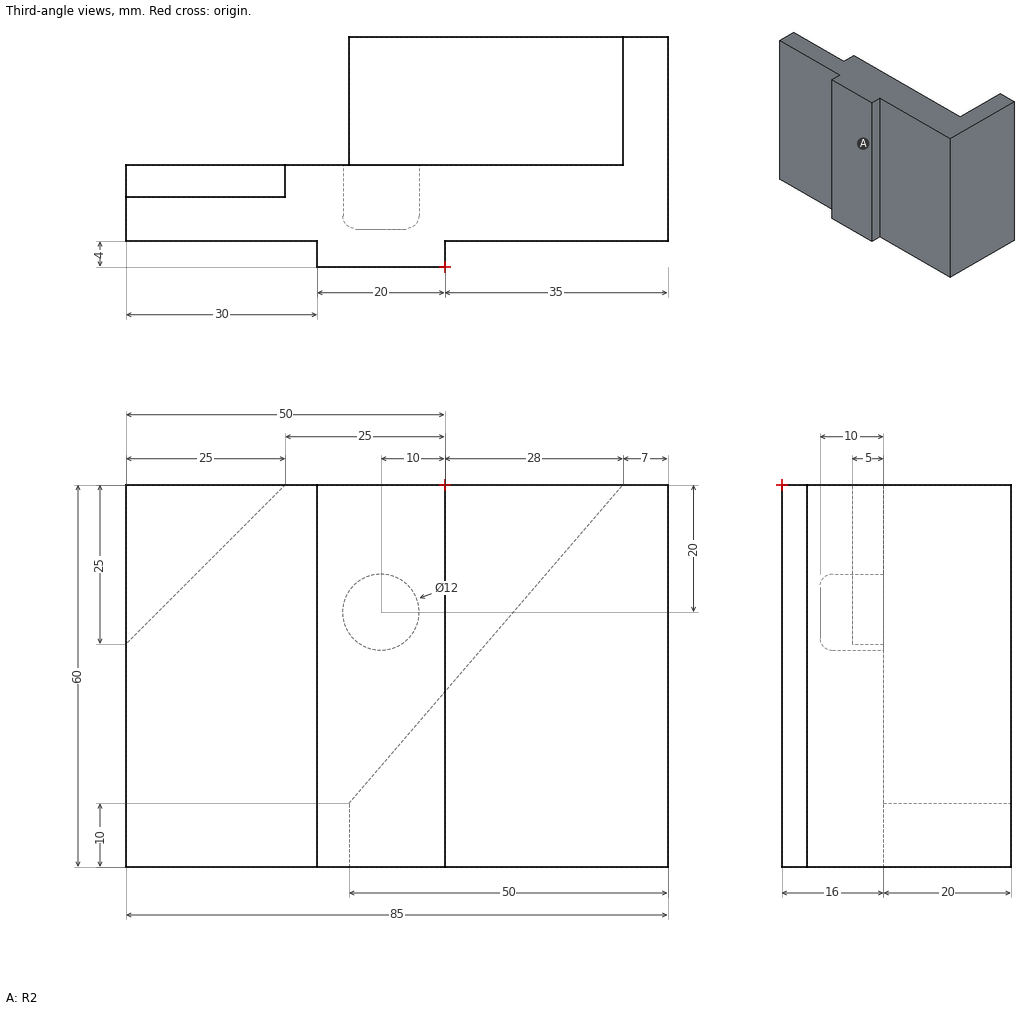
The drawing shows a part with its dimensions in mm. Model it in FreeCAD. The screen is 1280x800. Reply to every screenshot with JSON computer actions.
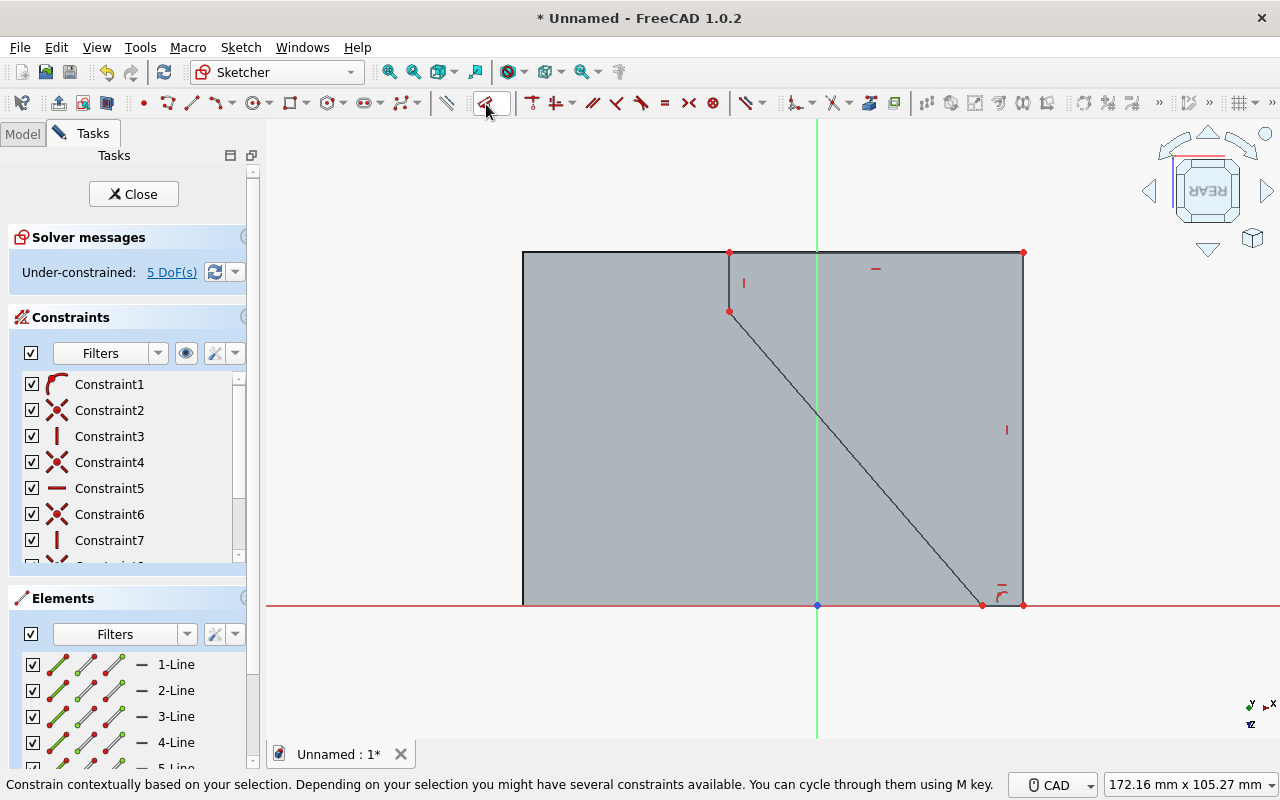
{"action": "left_click", "coordinate": [994, 606]}
{"action": "left_click", "coordinate": [1003, 640]}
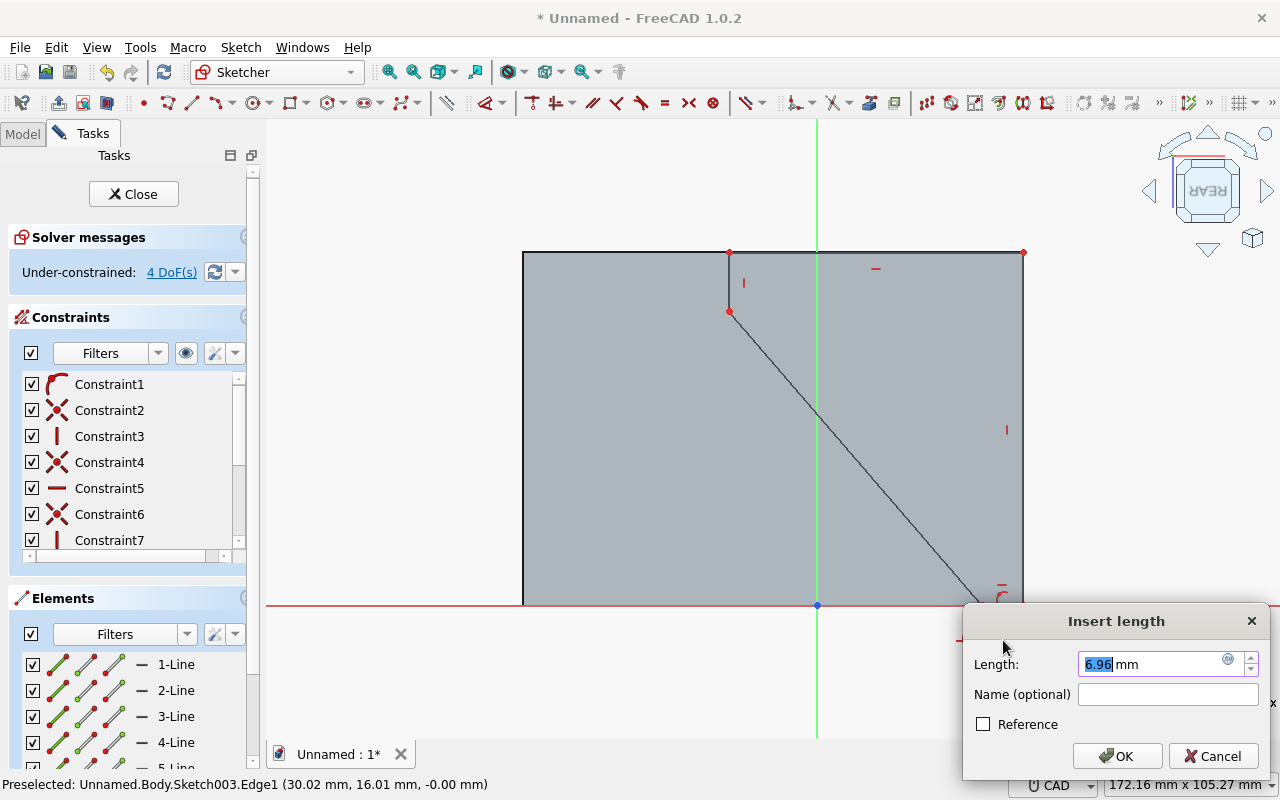
{"action": "type", "text": "7"}
{"action": "key", "text": "Return"}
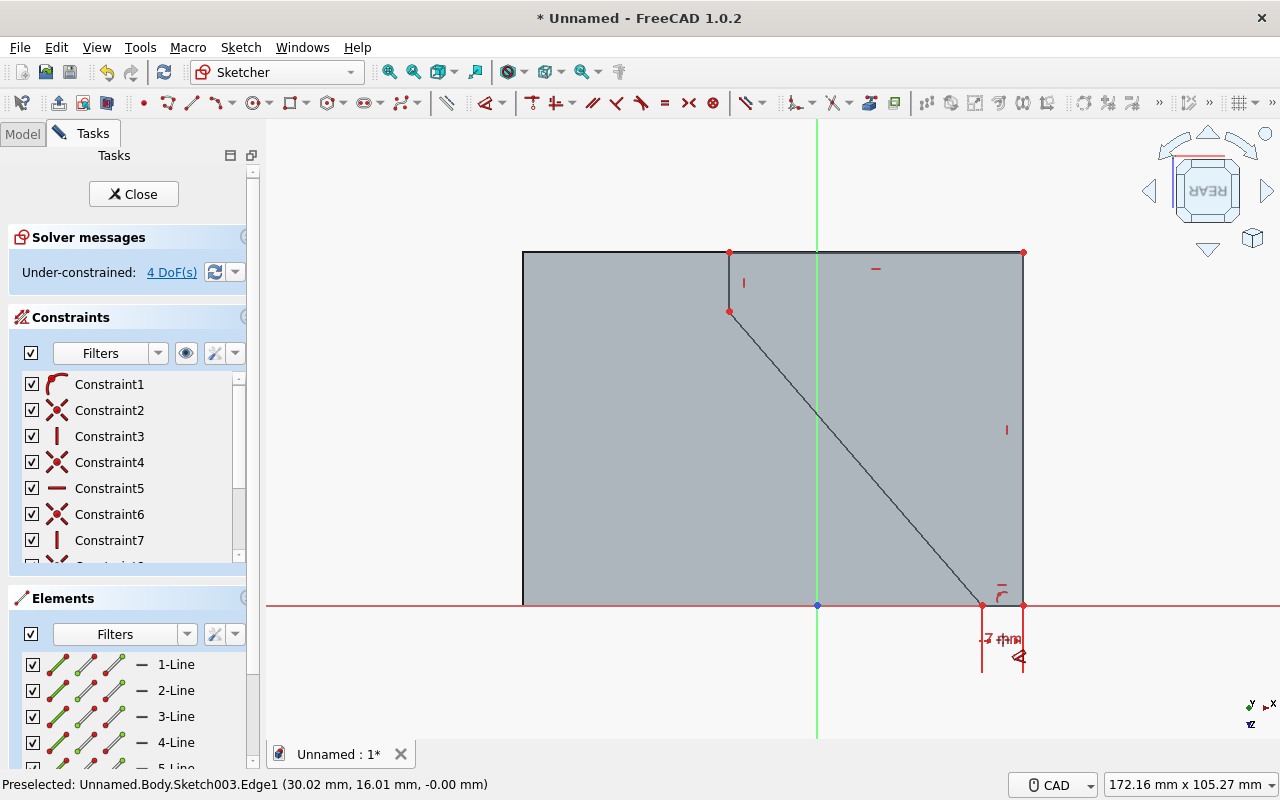
{"action": "left_click", "coordinate": [1023, 500]}
{"action": "left_click", "coordinate": [1057, 429]}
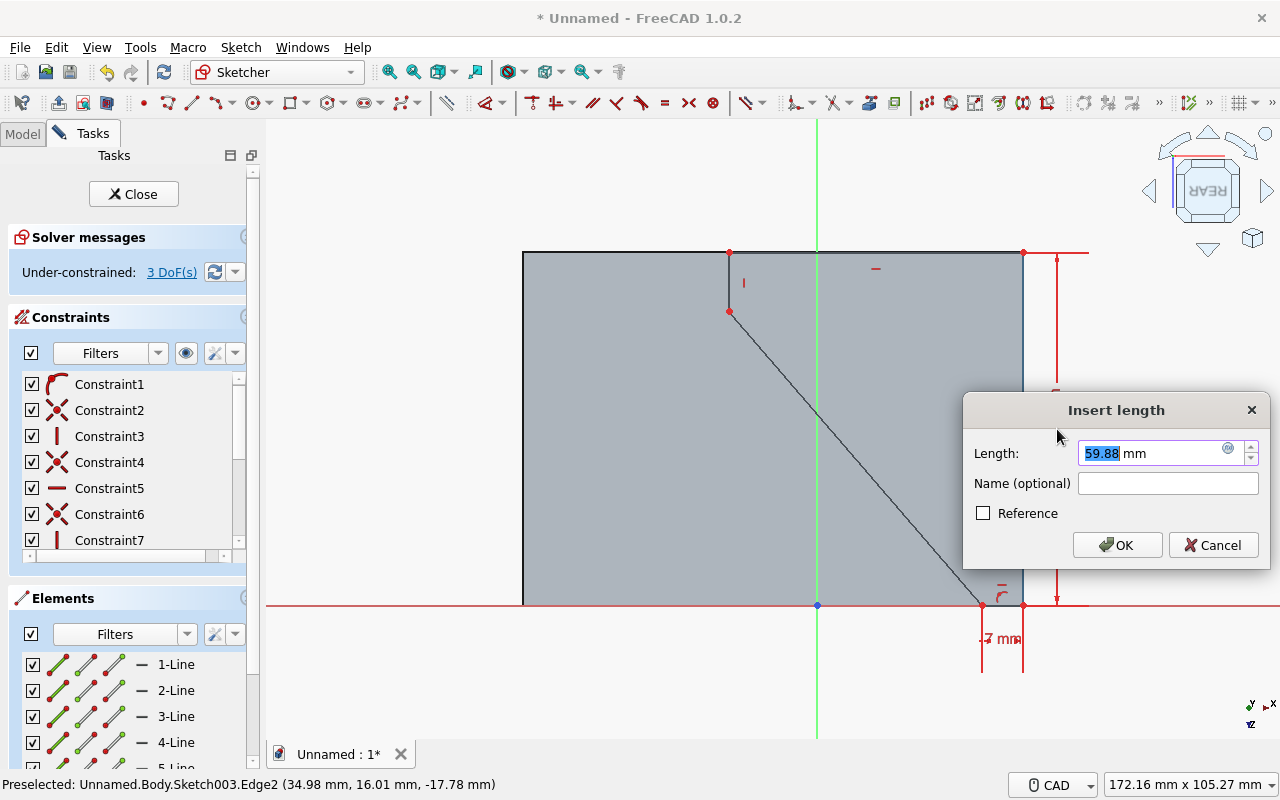
{"action": "type", "text": "60"}
{"action": "key", "text": "Return"}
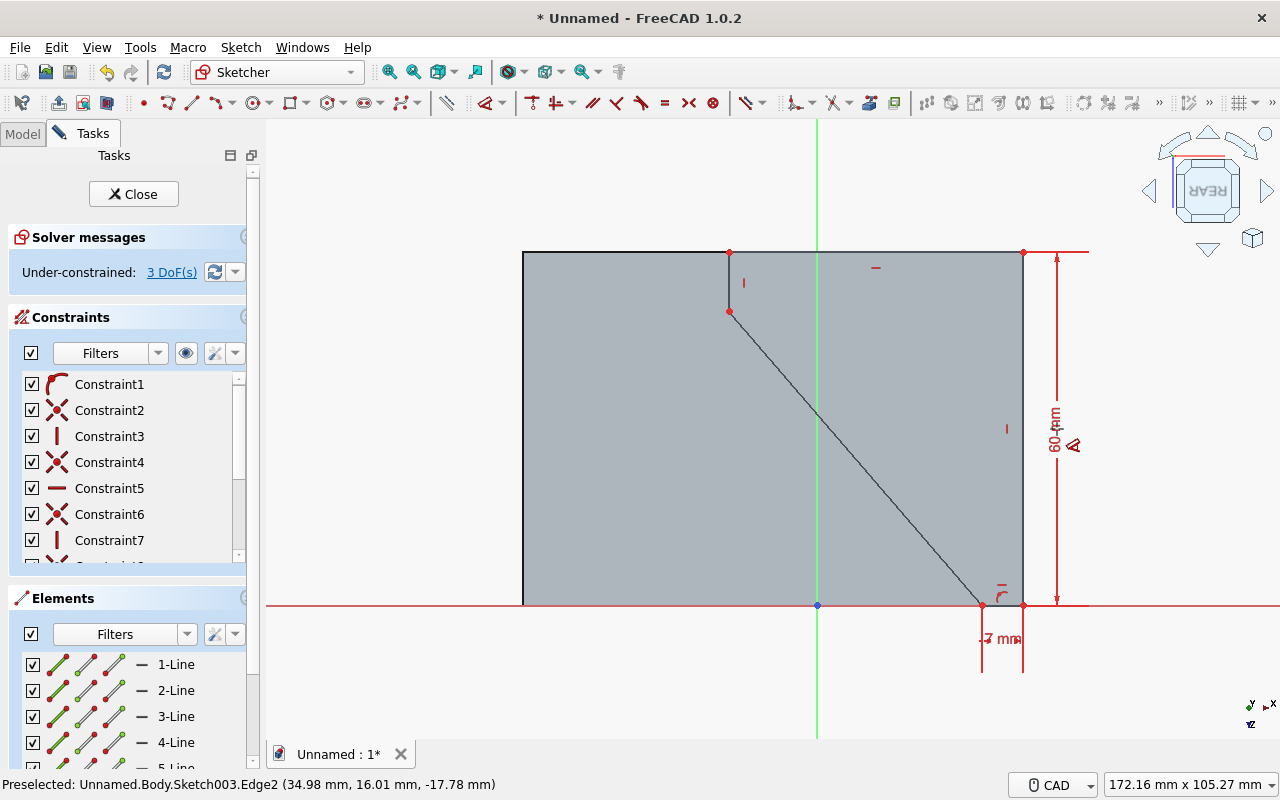
{"action": "left_click", "coordinate": [935, 252]}
{"action": "left_click", "coordinate": [876, 218]}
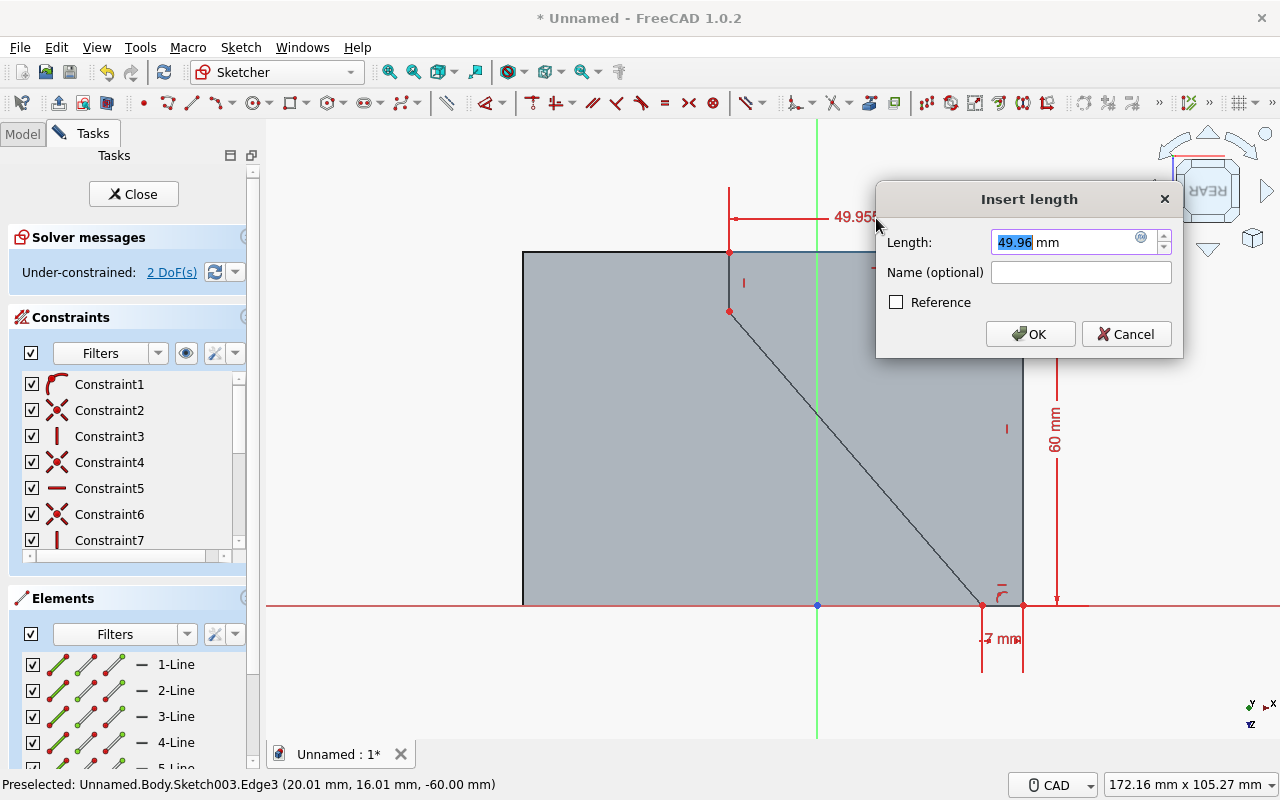
{"action": "type", "text": "50"}
{"action": "key", "text": "Return"}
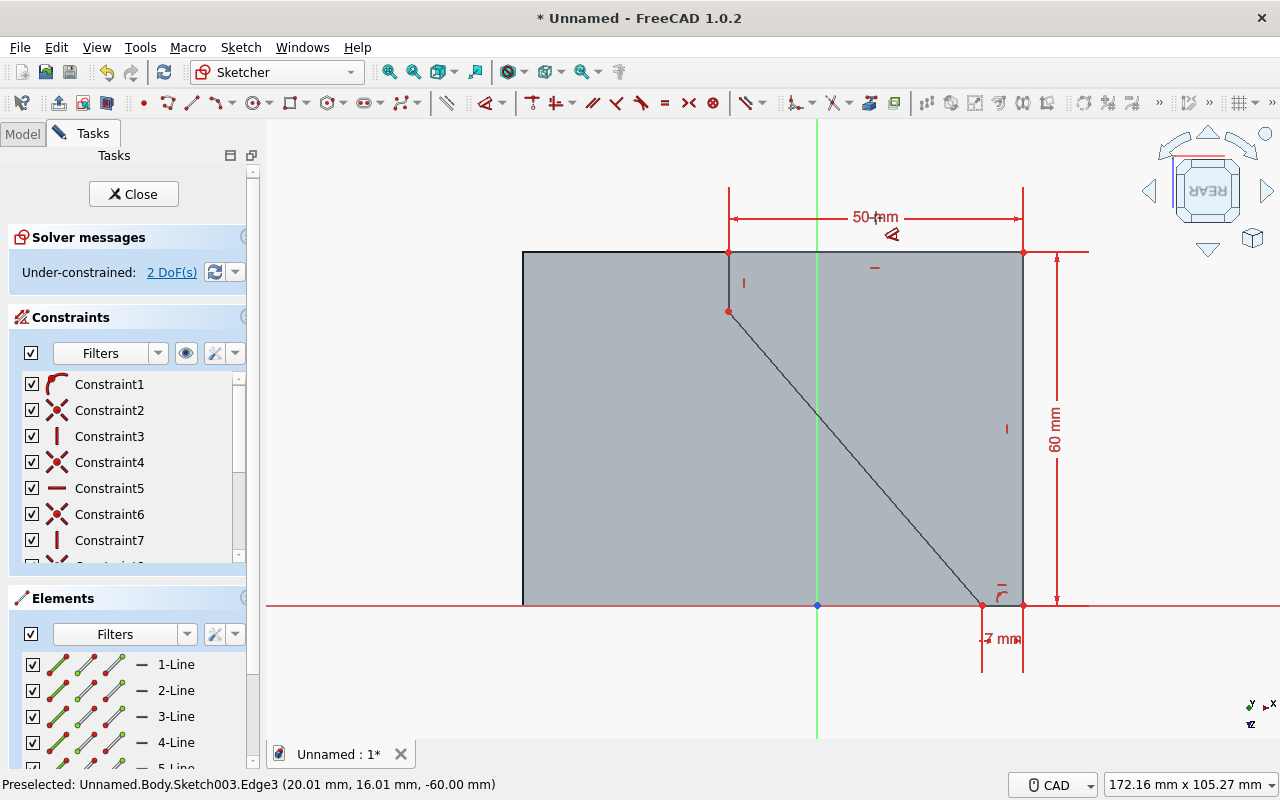
{"action": "left_click", "coordinate": [729, 270]}
{"action": "left_click", "coordinate": [695, 282]}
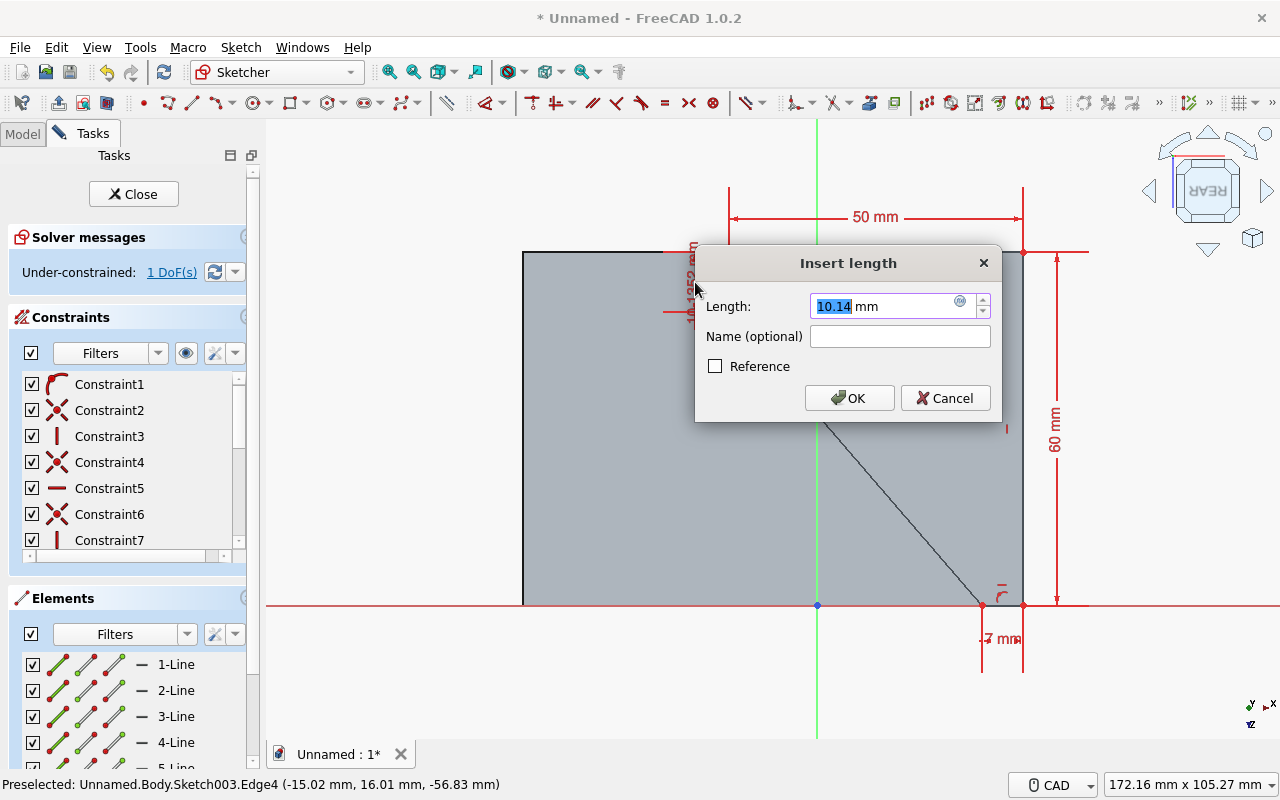
{"action": "type", "text": "10"}
{"action": "key", "text": "Return"}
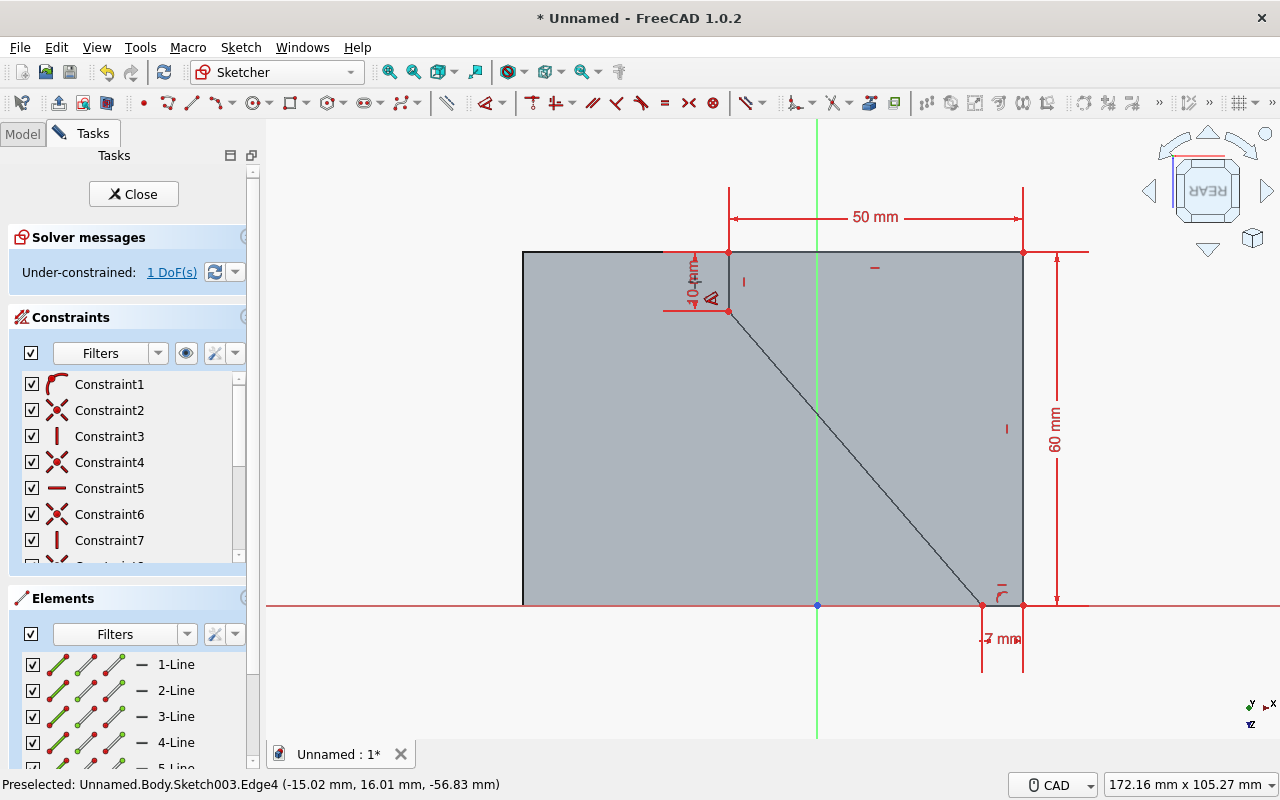
{"action": "left_click", "coordinate": [982, 606]}
{"action": "left_click", "coordinate": [900, 640]}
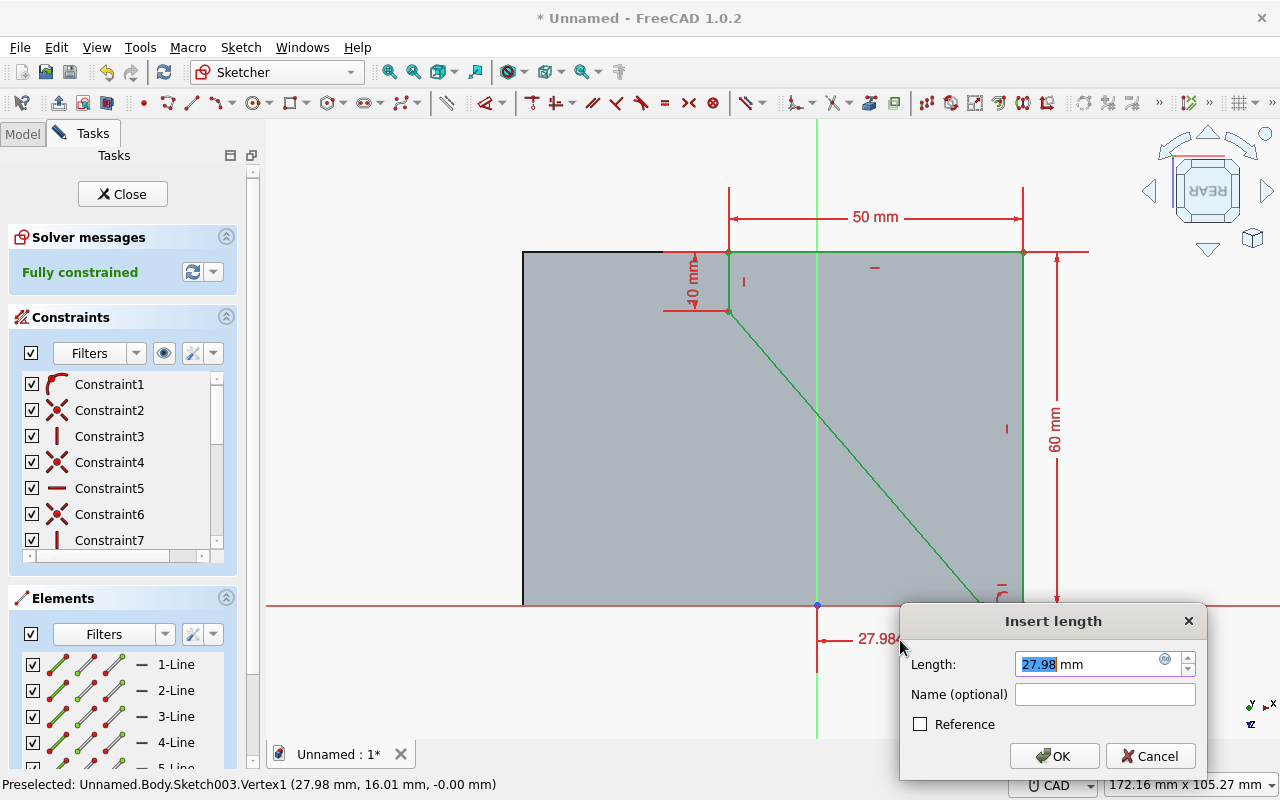
{"action": "type", "text": "28"}
{"action": "key", "text": "Return"}
{"action": "key", "text": "Escape"}